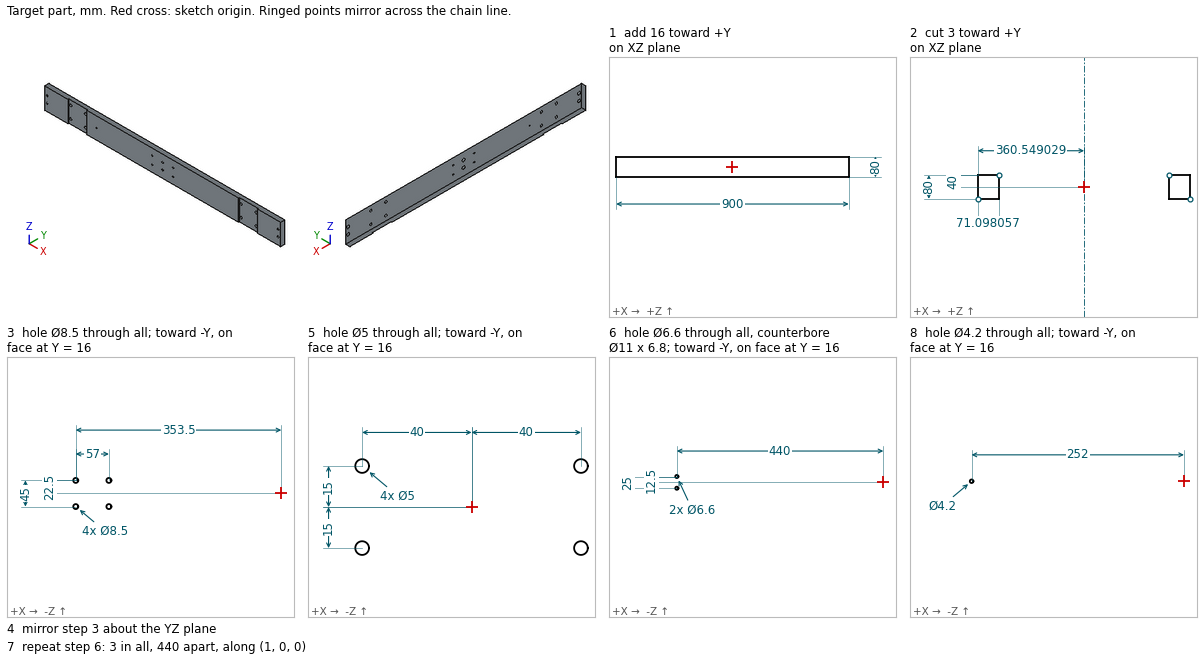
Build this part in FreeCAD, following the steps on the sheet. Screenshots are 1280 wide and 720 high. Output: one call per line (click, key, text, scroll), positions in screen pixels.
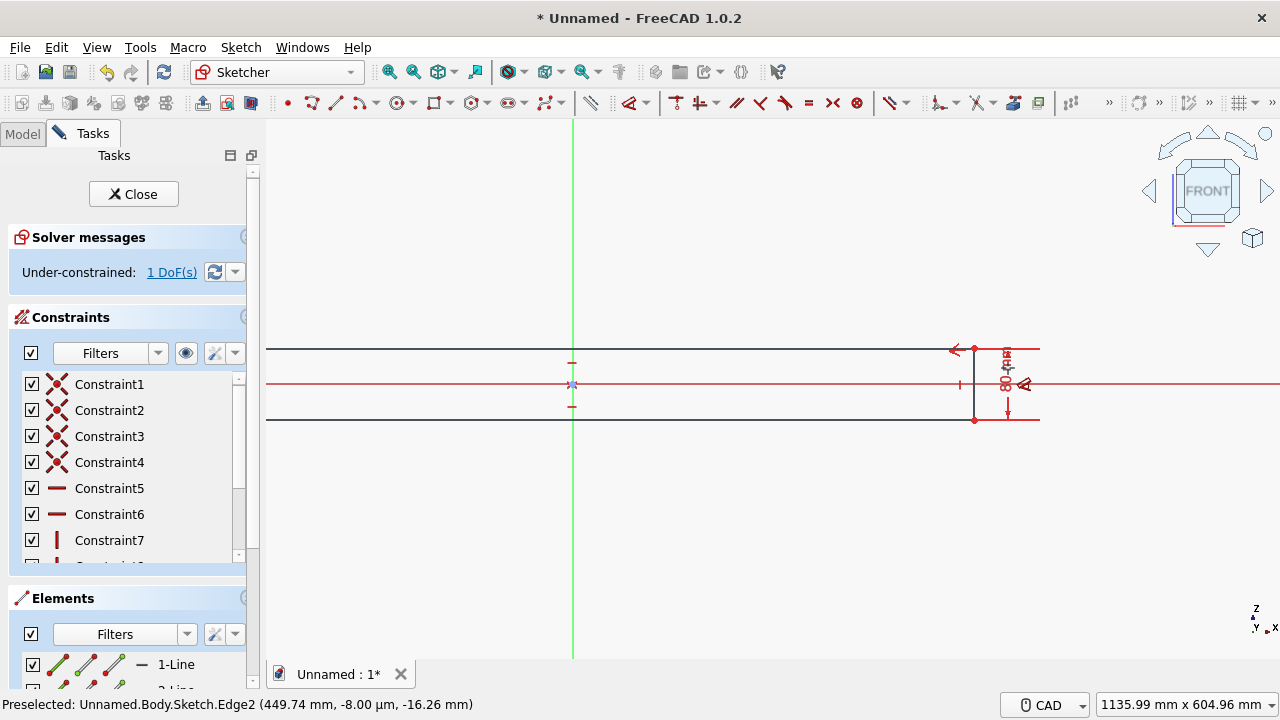
click(412, 420)
click(634, 454)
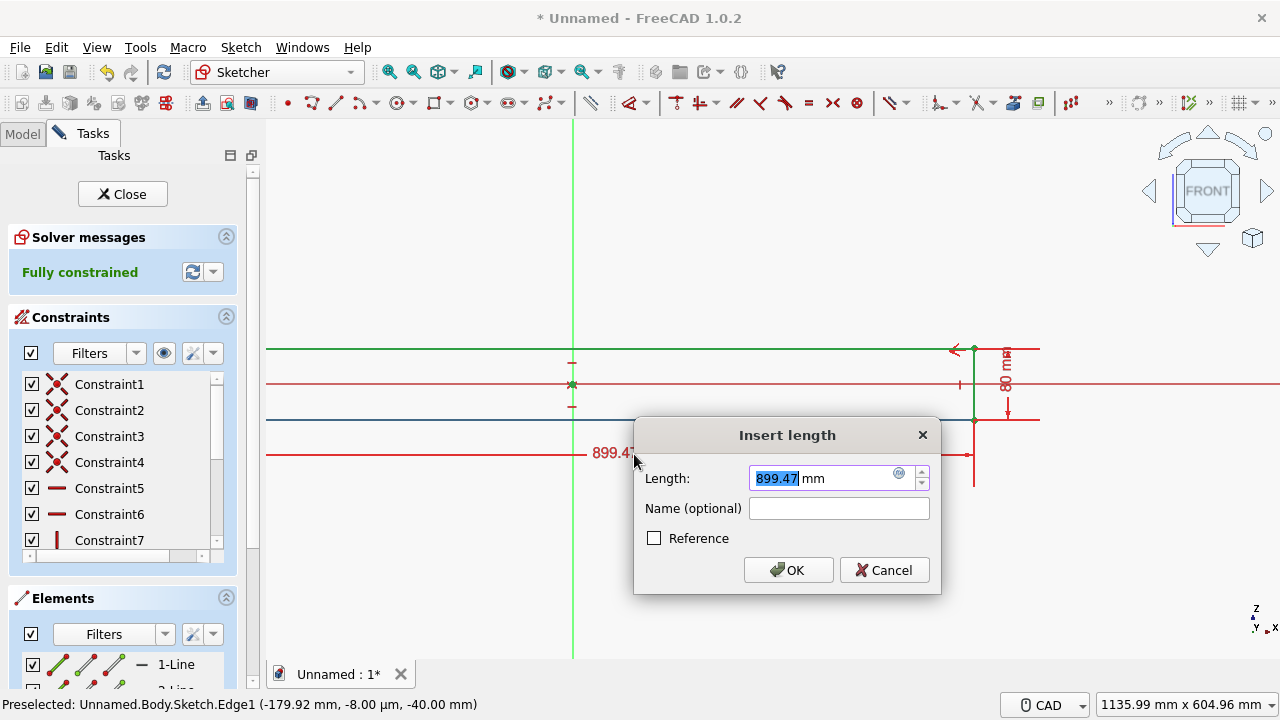
text(900)
key(Return)
key(Escape)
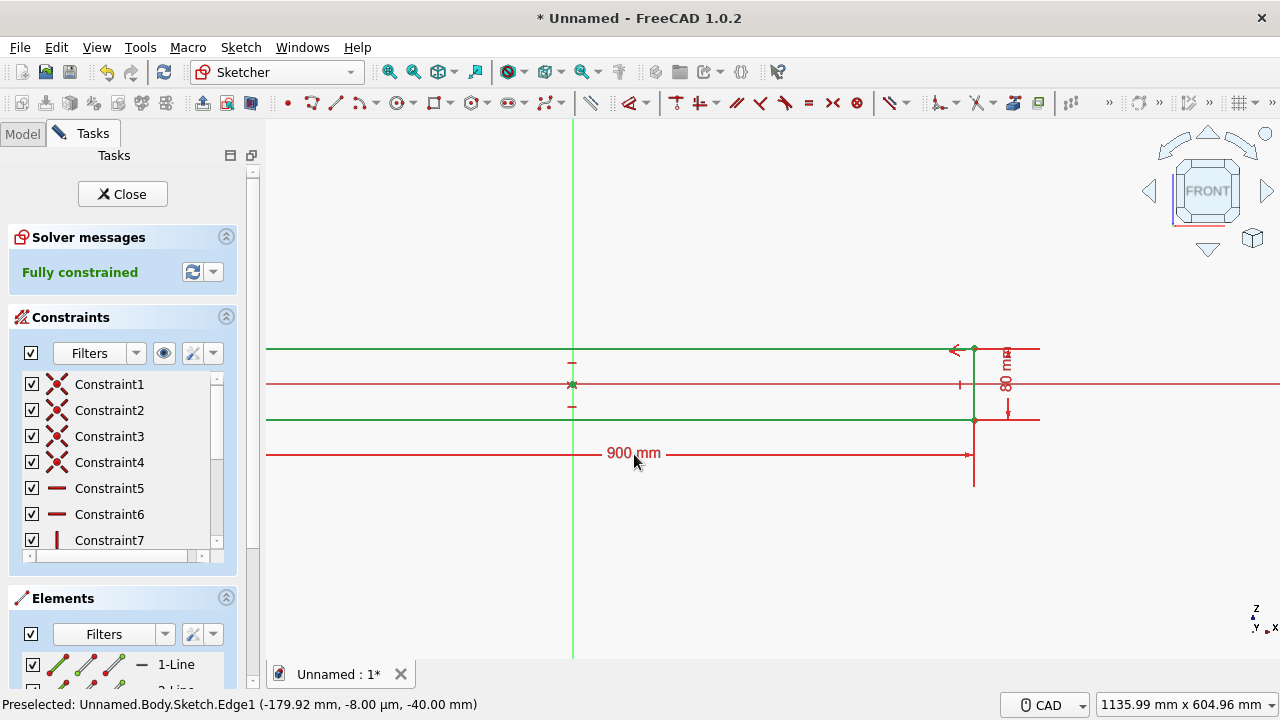
click(123, 194)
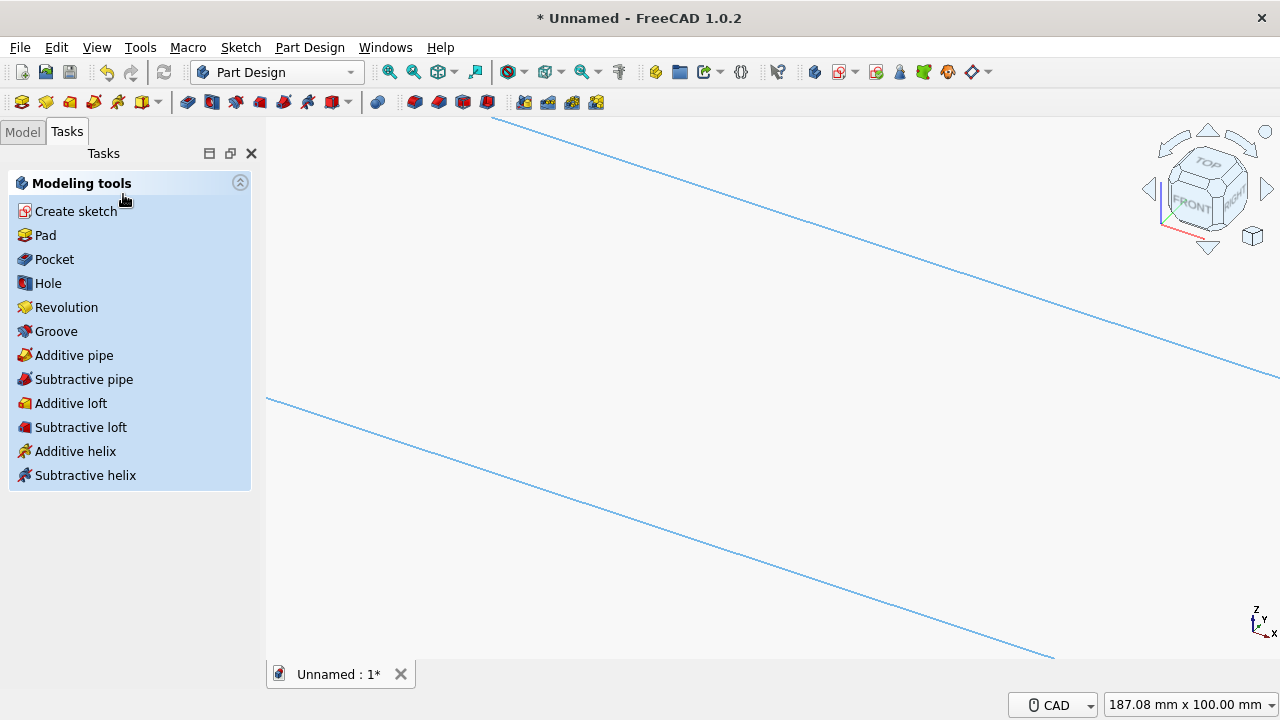
click(22, 102)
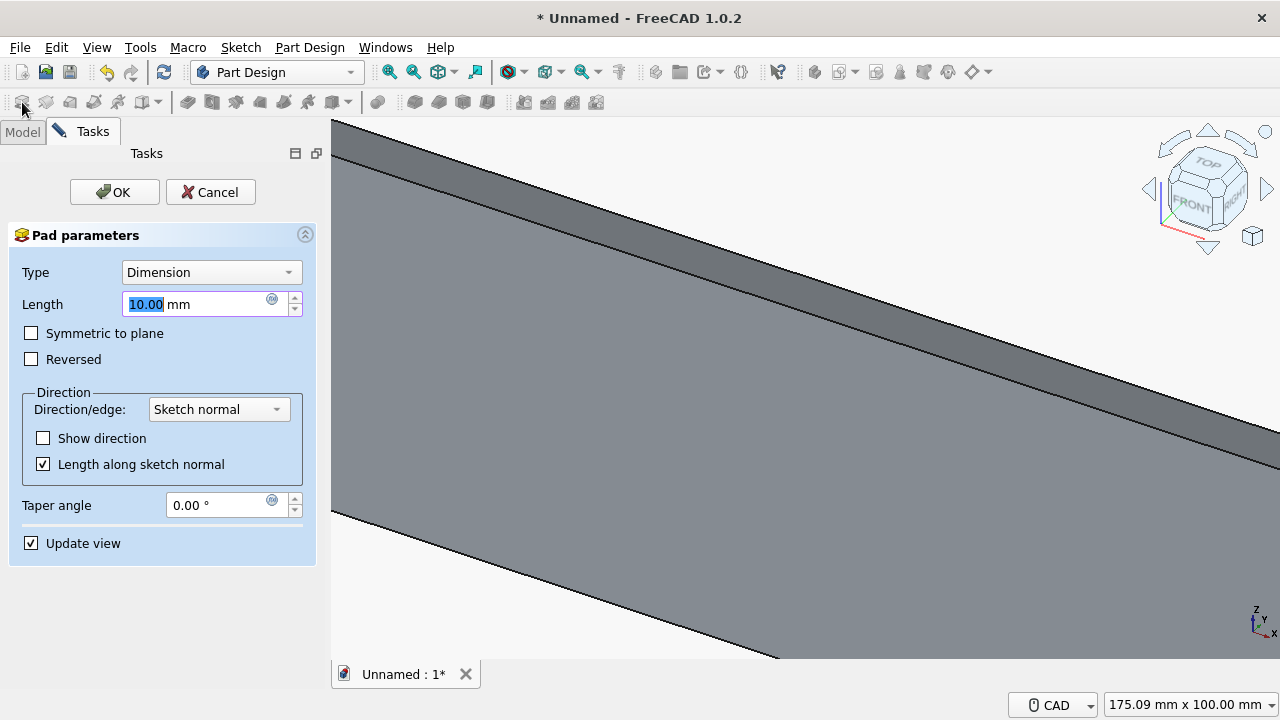
text(16)
key(Tab)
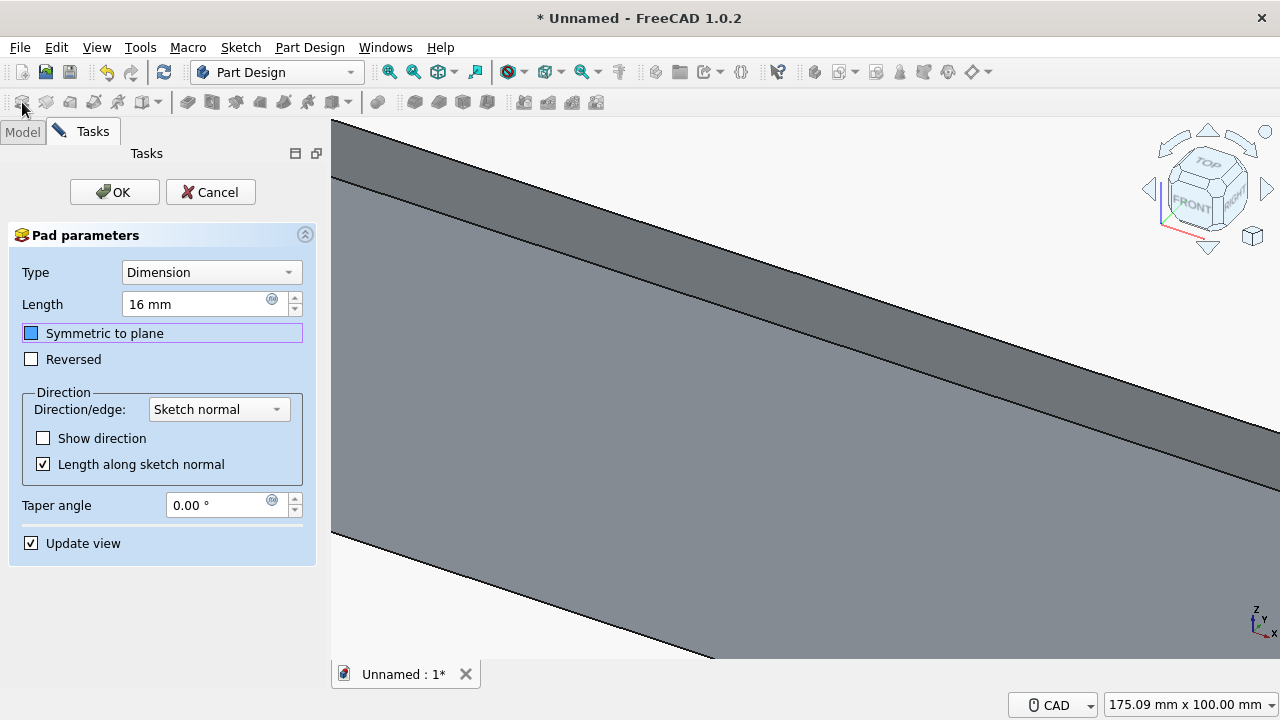
click(30, 359)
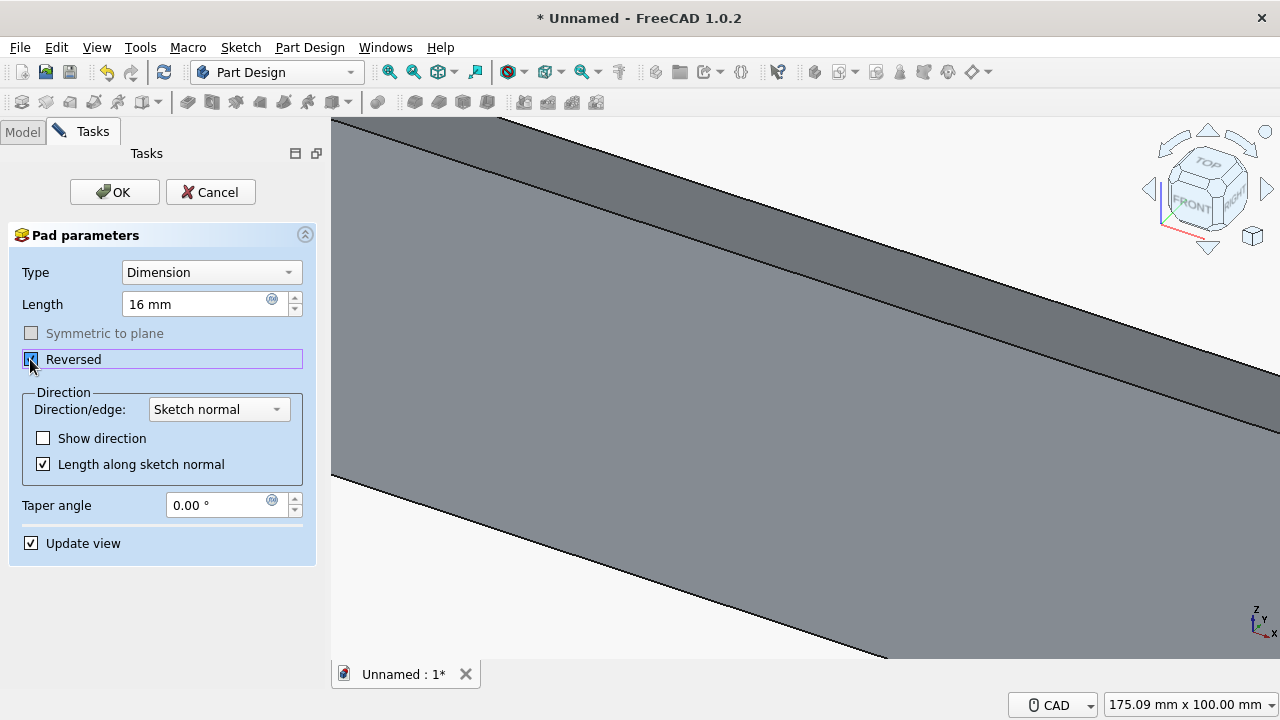
click(115, 192)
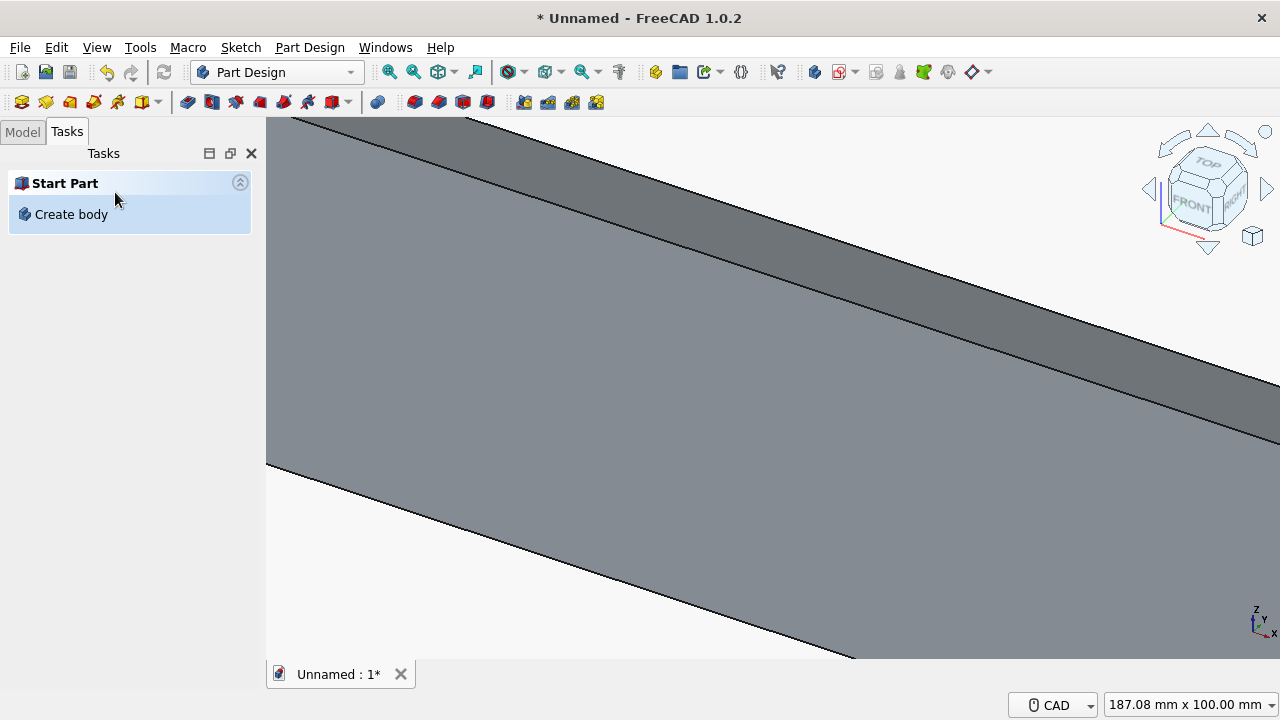
click(390, 72)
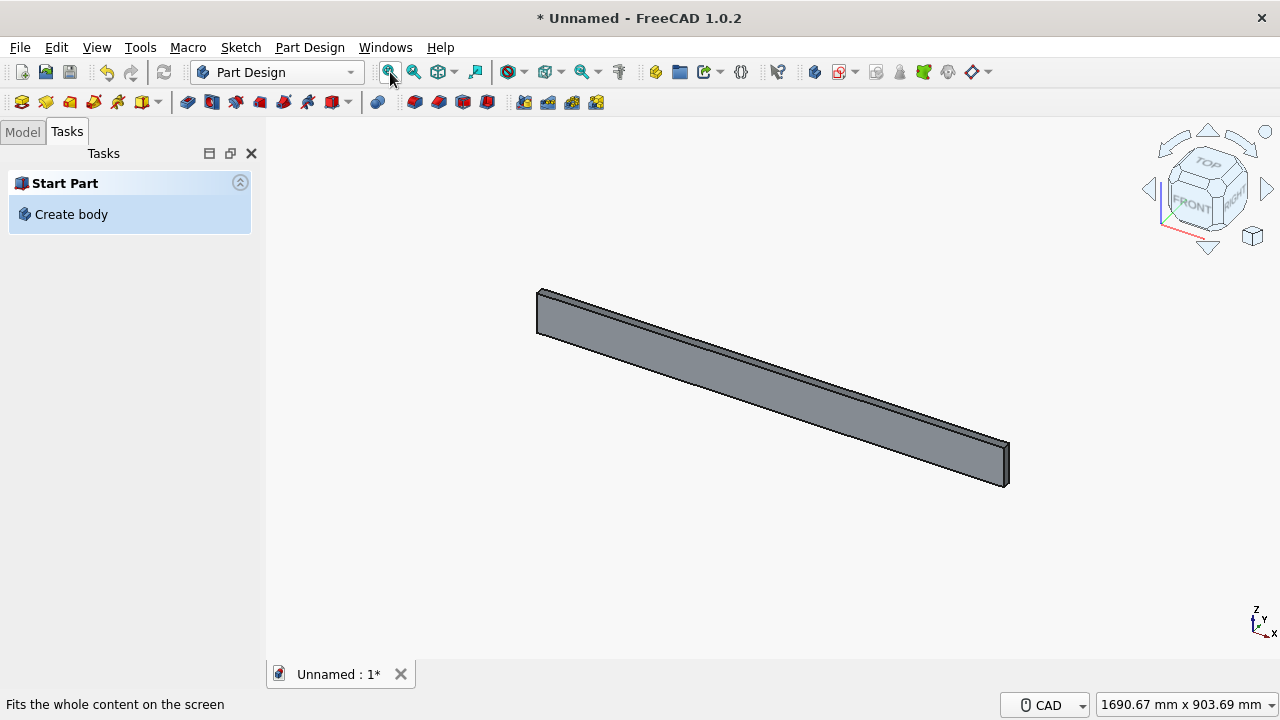
click(840, 72)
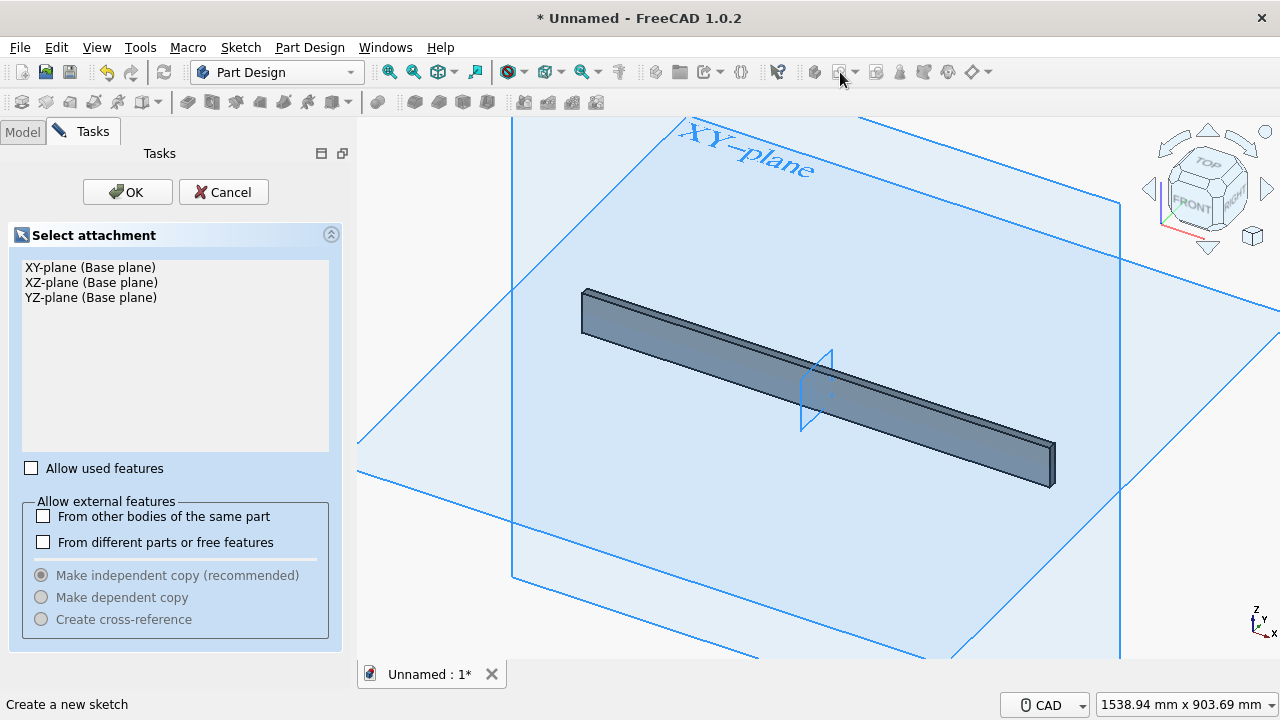
click(82, 282)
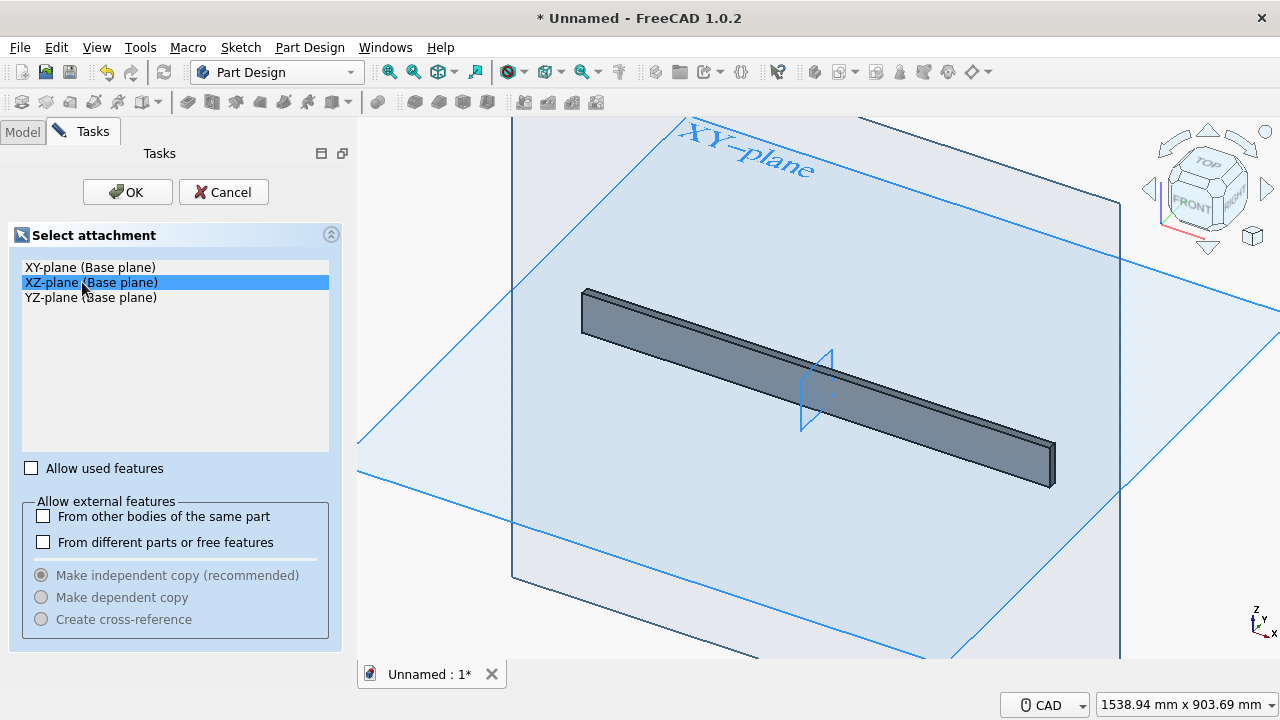
click(128, 192)